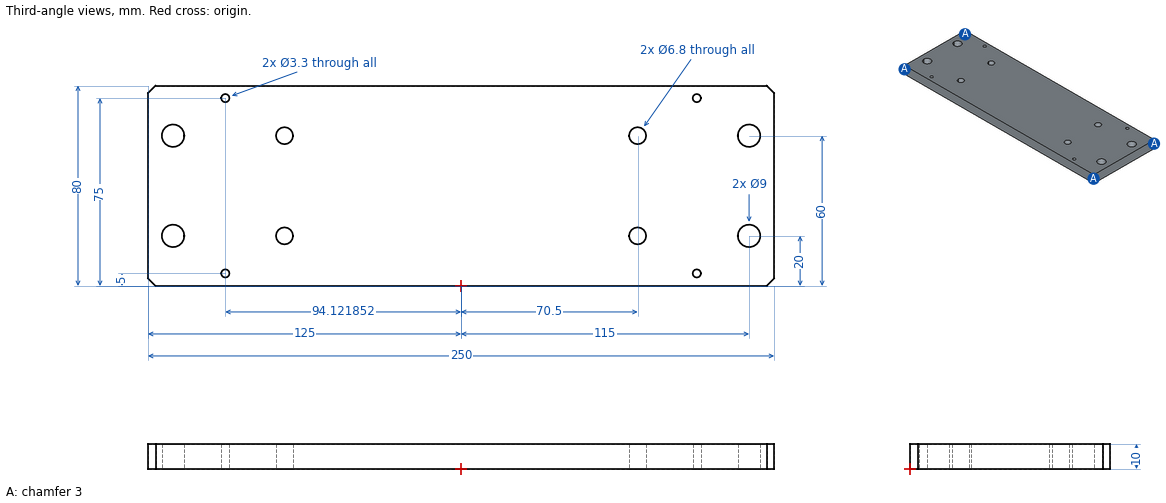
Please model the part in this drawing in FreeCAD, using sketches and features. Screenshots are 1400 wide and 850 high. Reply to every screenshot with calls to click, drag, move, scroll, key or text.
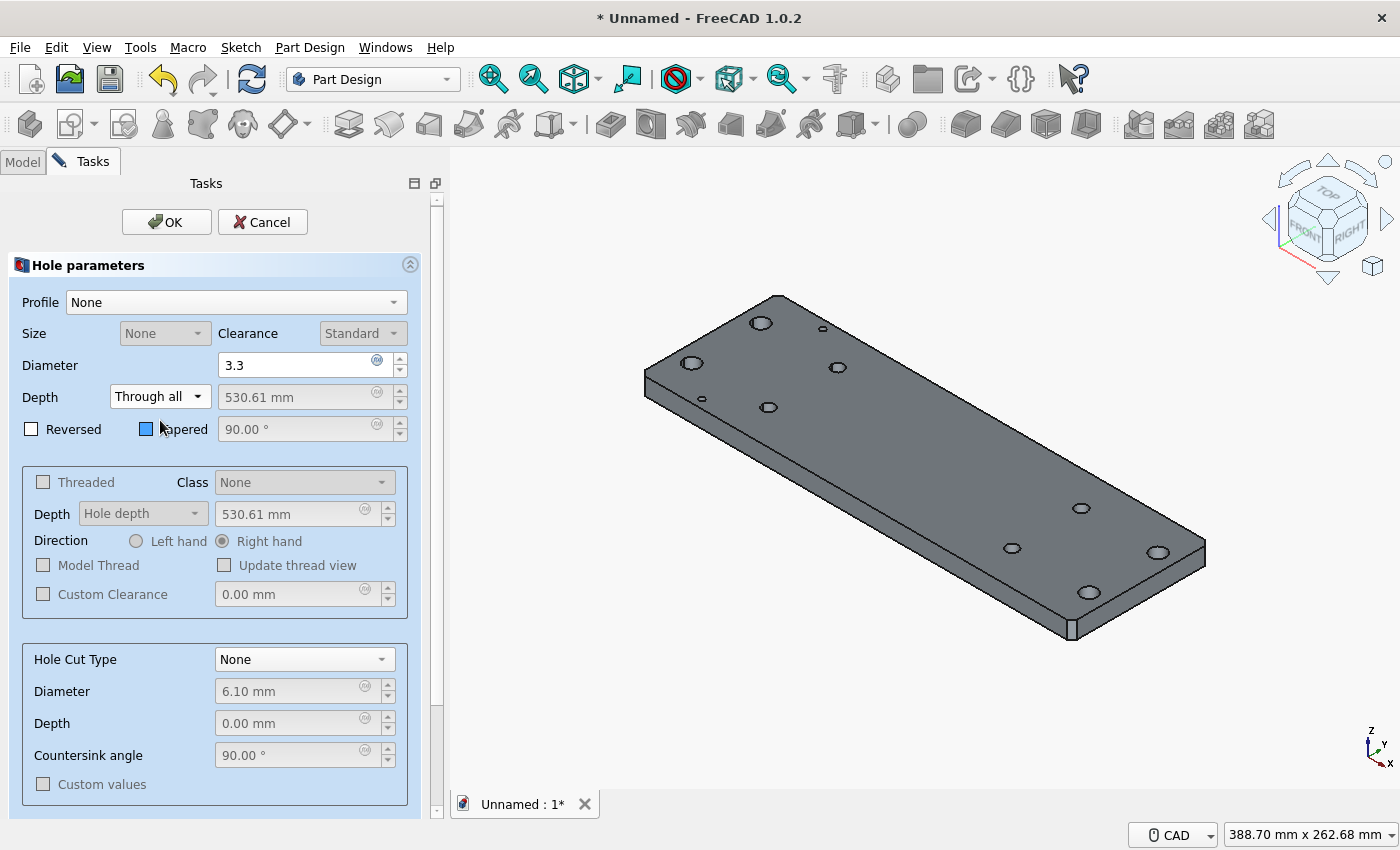
click(167, 222)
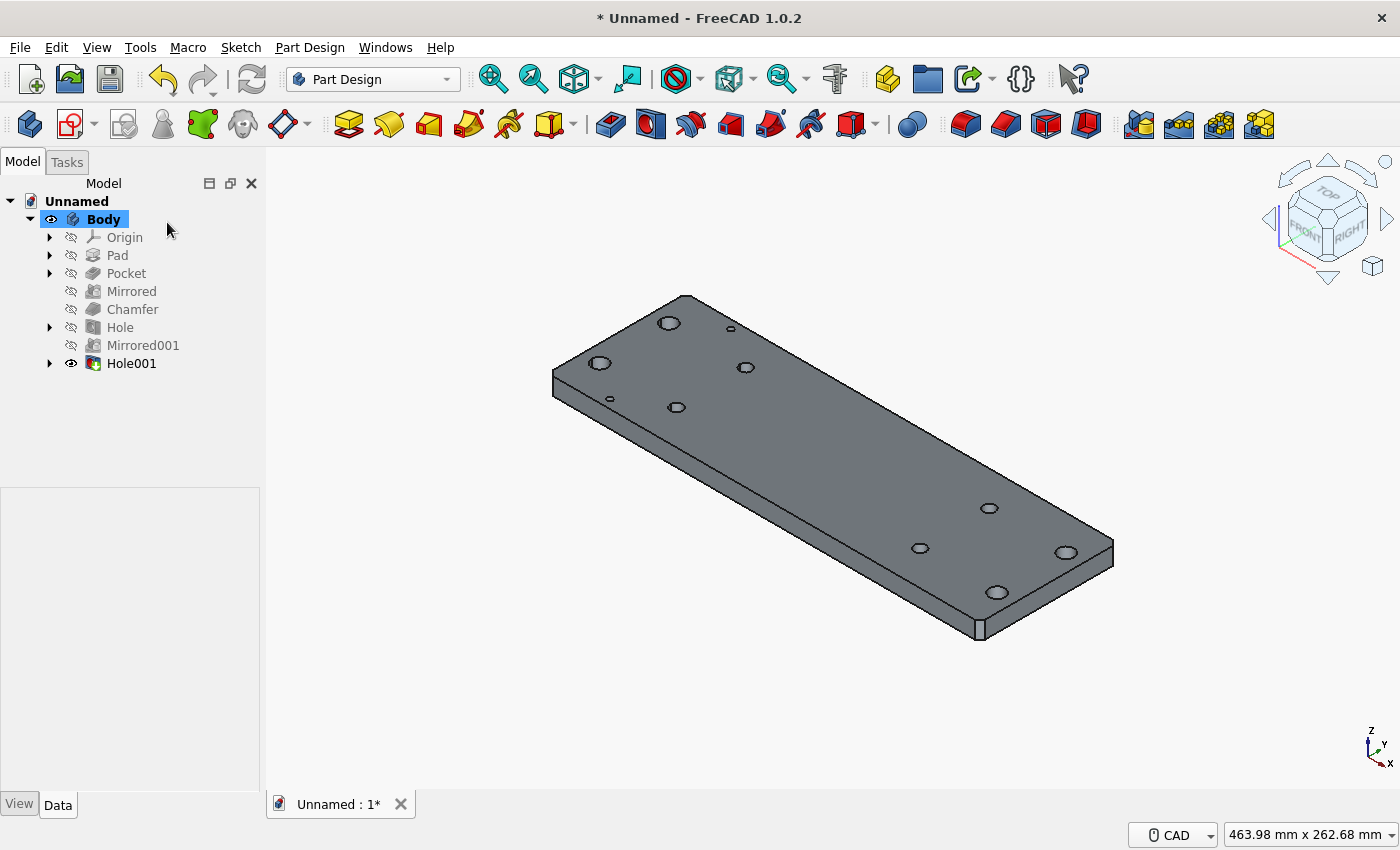
click(116, 363)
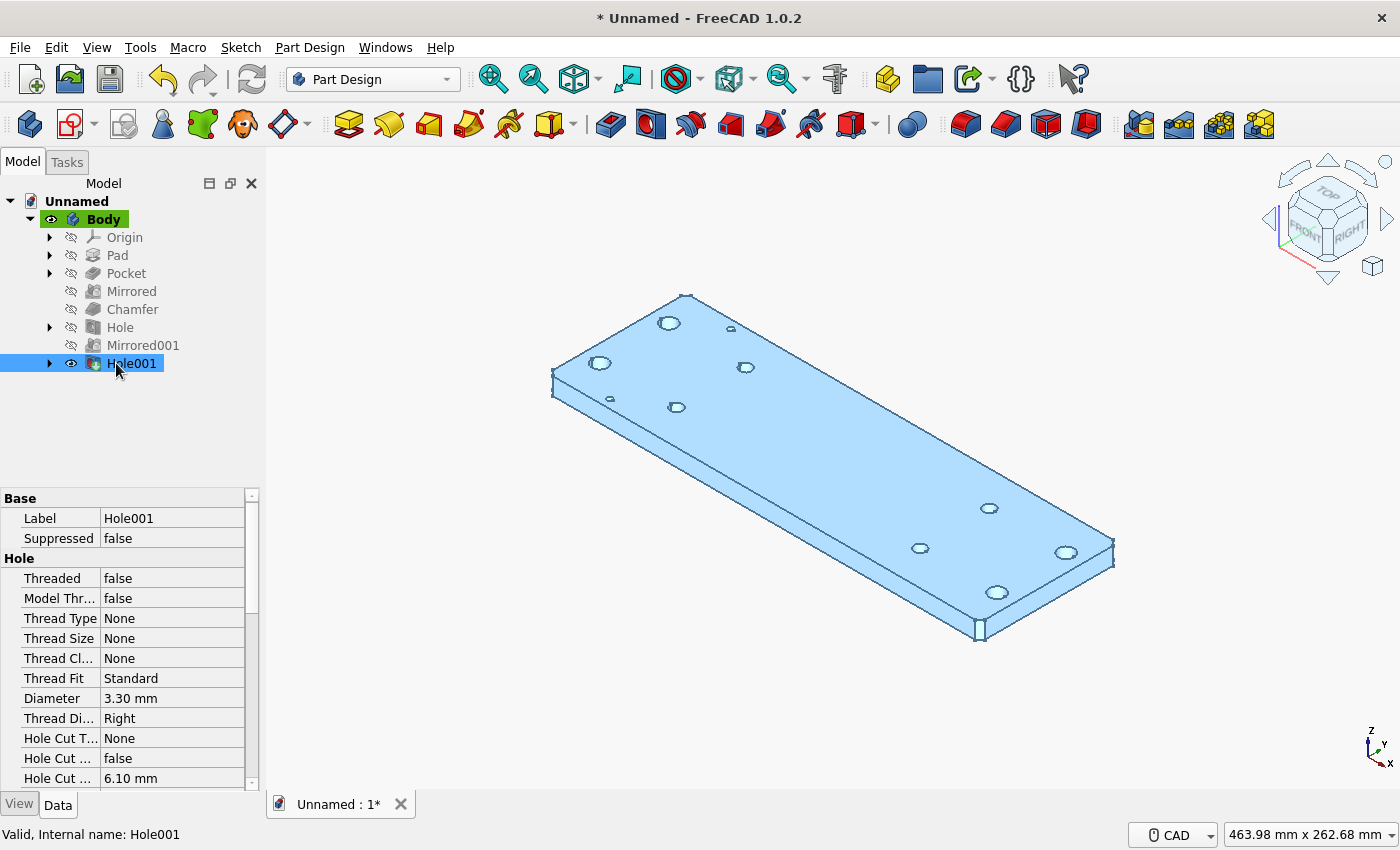
click(1140, 124)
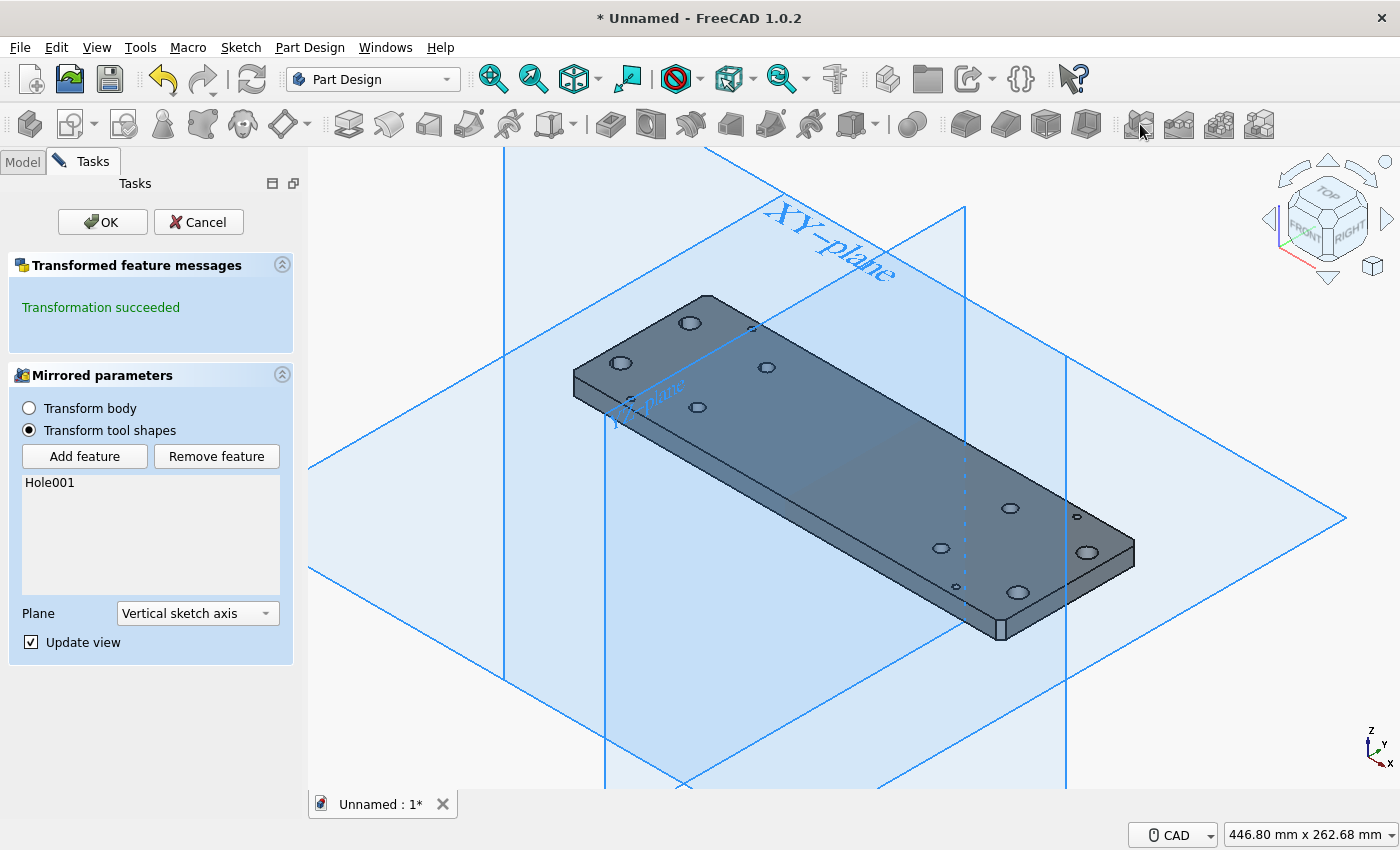
click(198, 614)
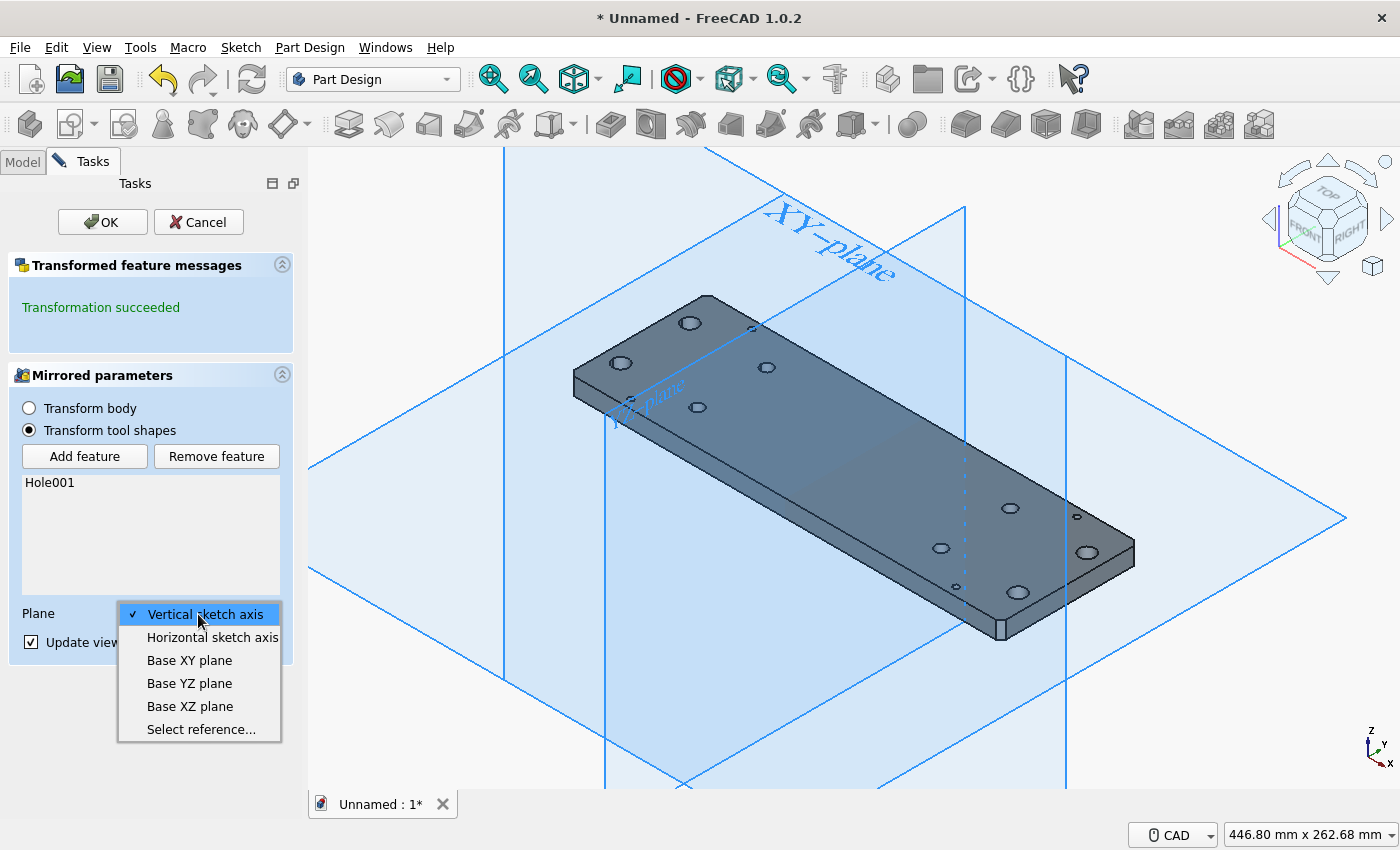
click(198, 684)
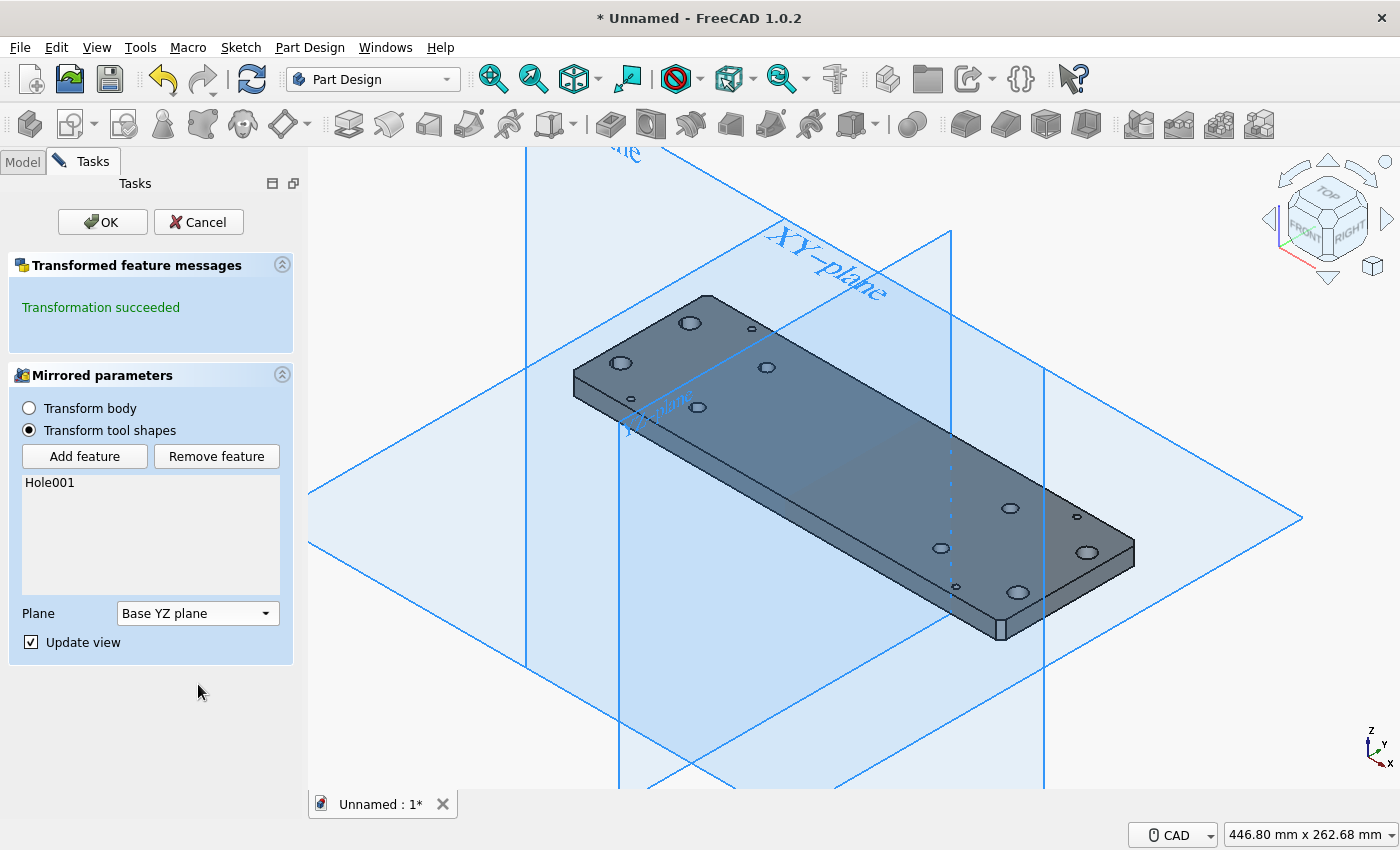
click(103, 222)